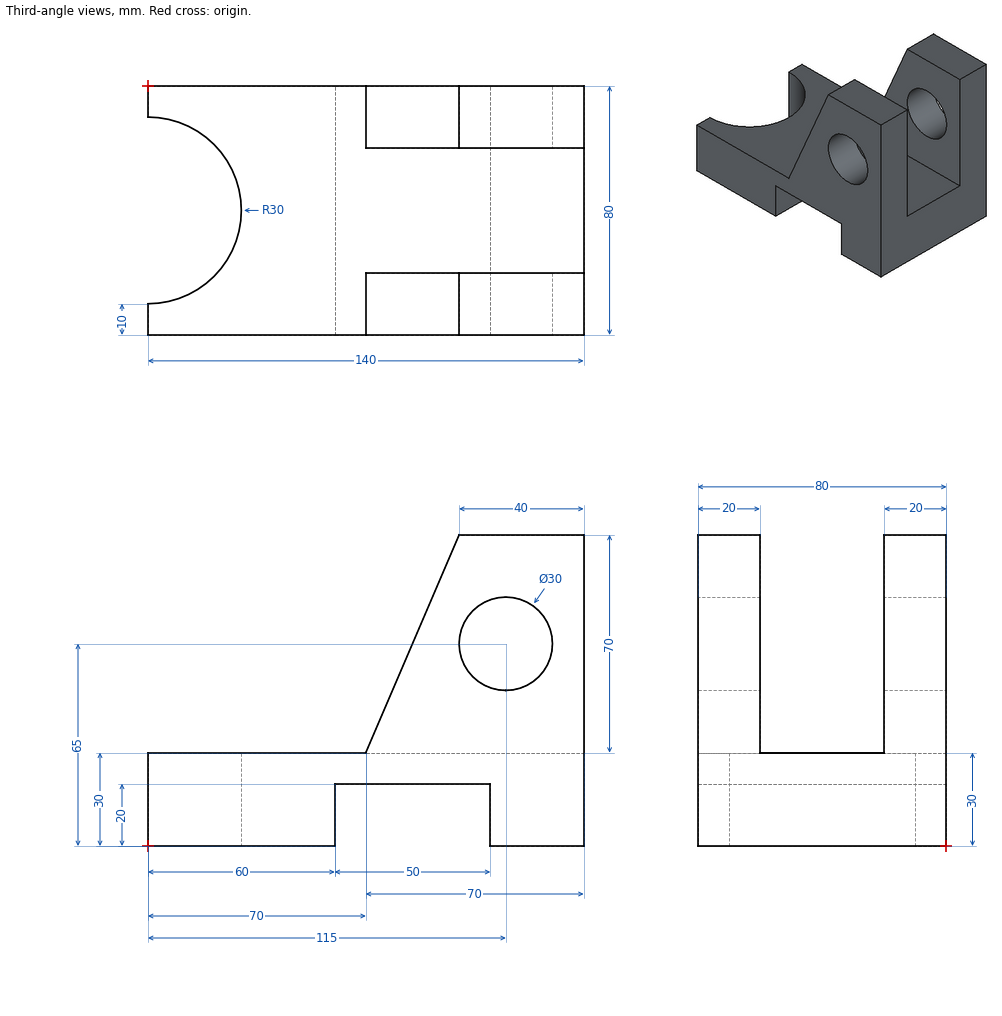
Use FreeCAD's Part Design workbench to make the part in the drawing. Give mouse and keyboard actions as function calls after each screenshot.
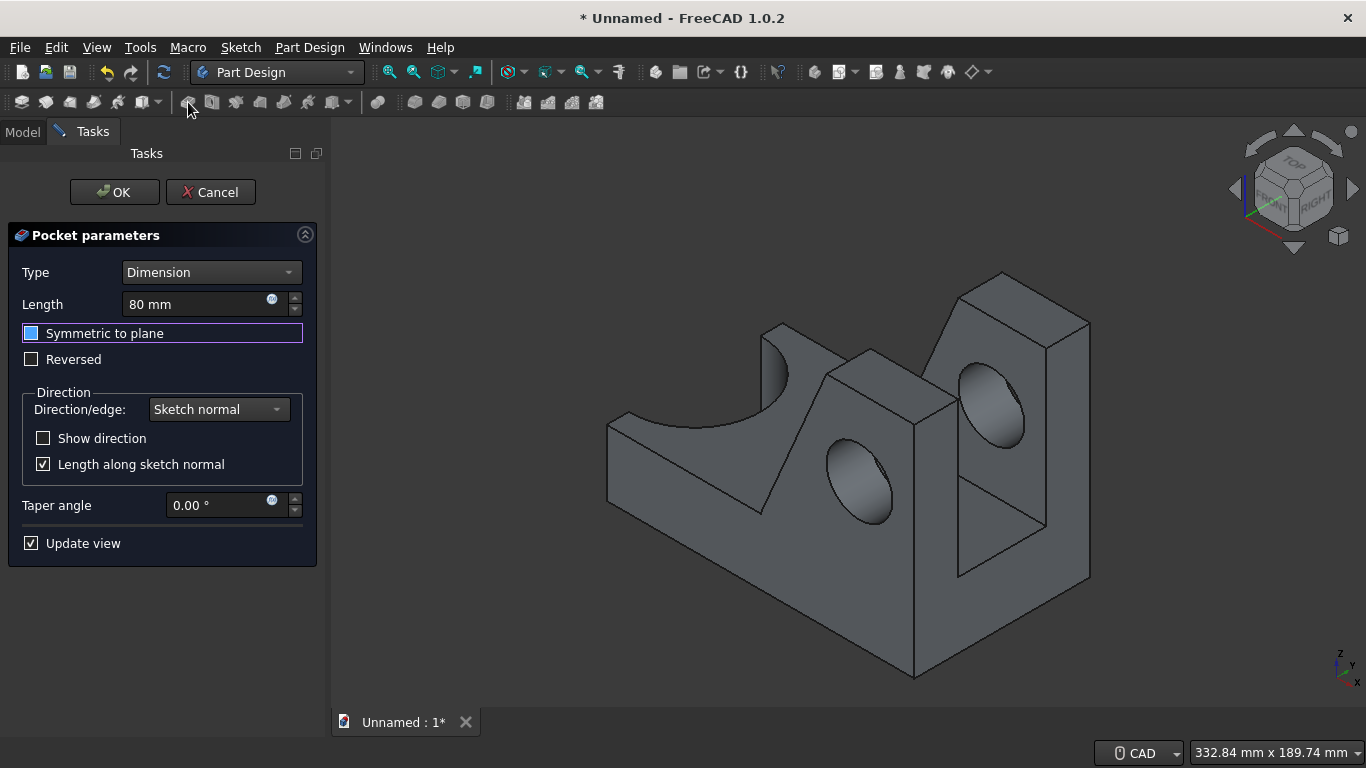
click(115, 192)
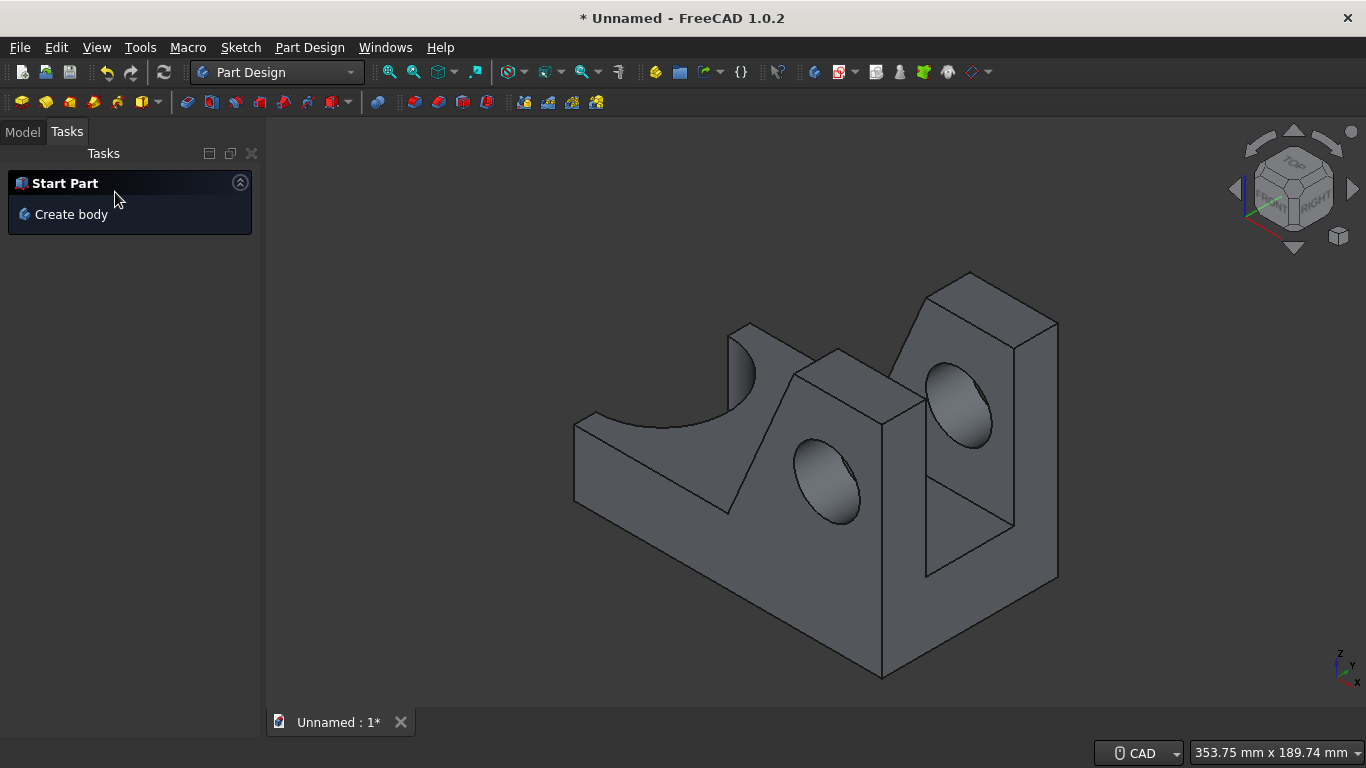
click(816, 585)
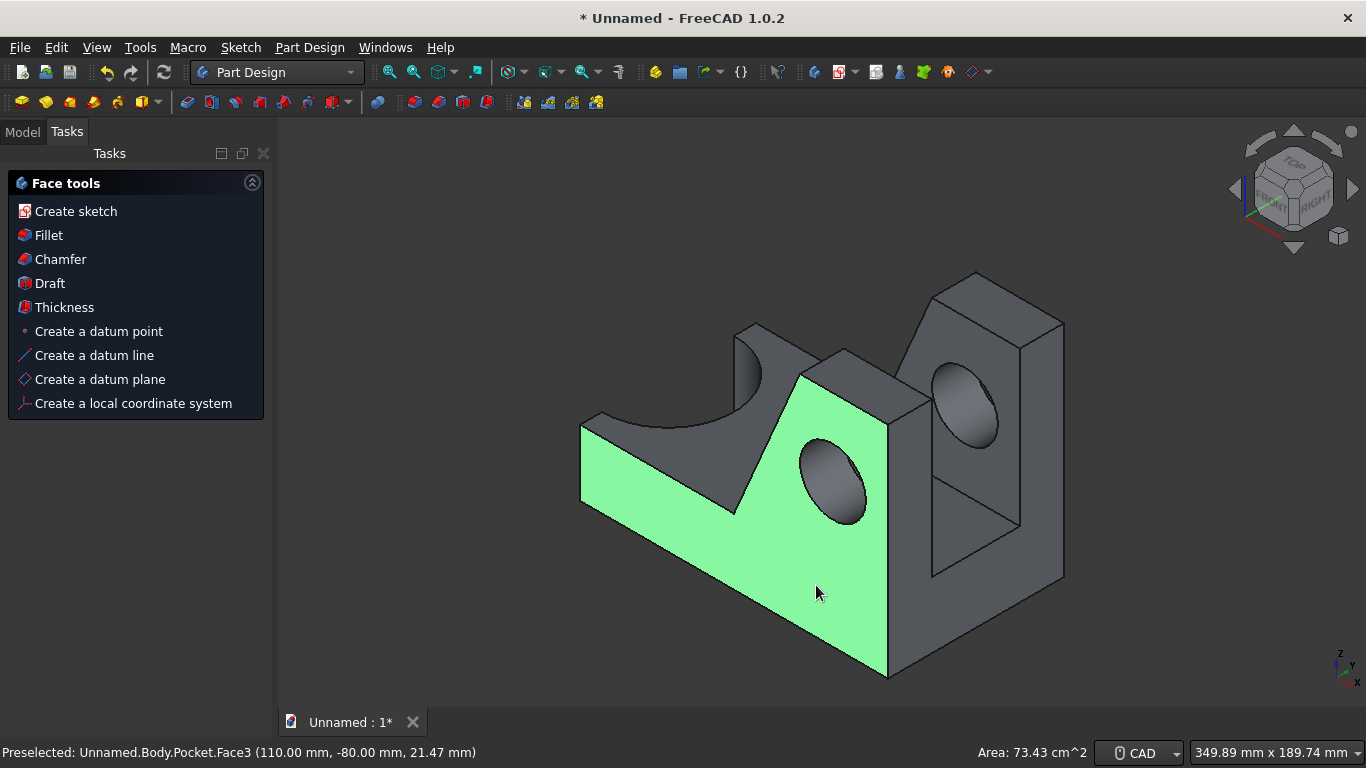
click(840, 72)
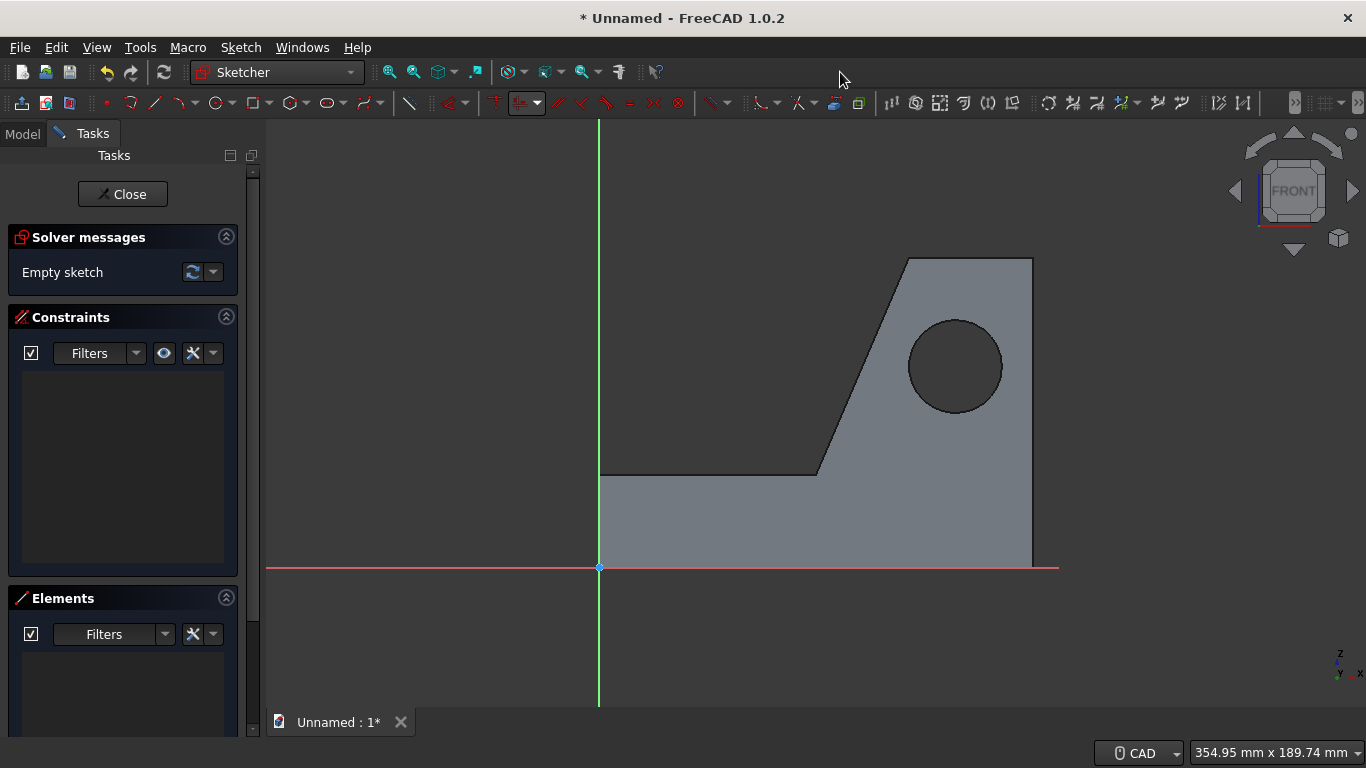
scroll(796, 679, up, 3)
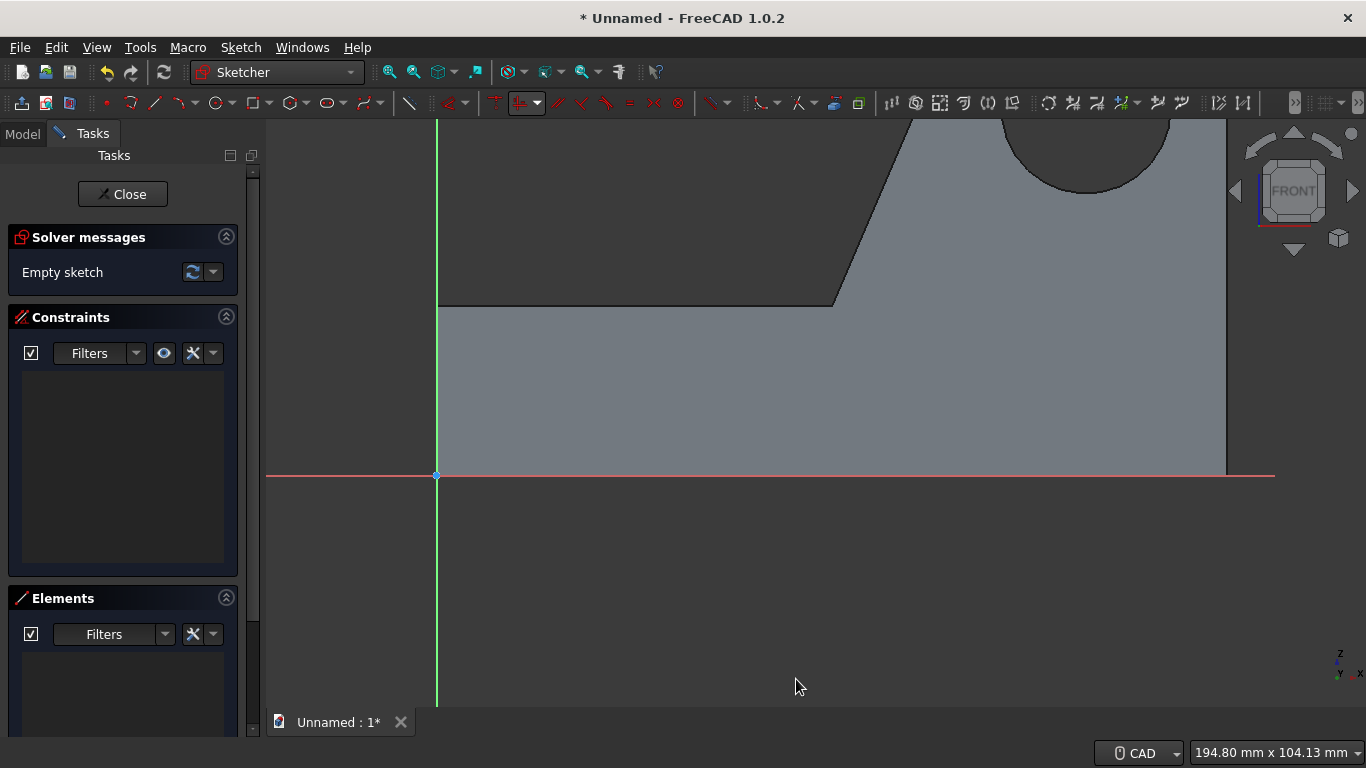
click(254, 104)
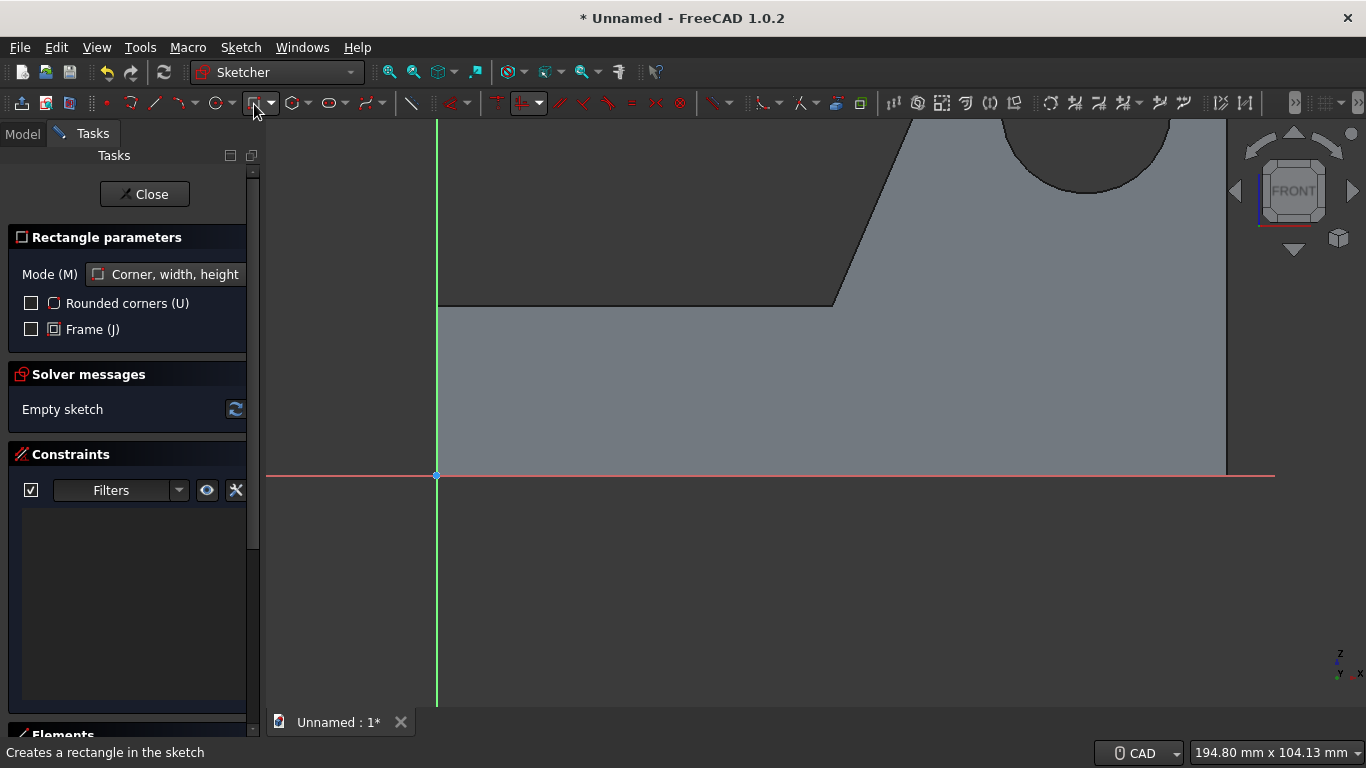
click(776, 363)
click(1058, 476)
key(Escape)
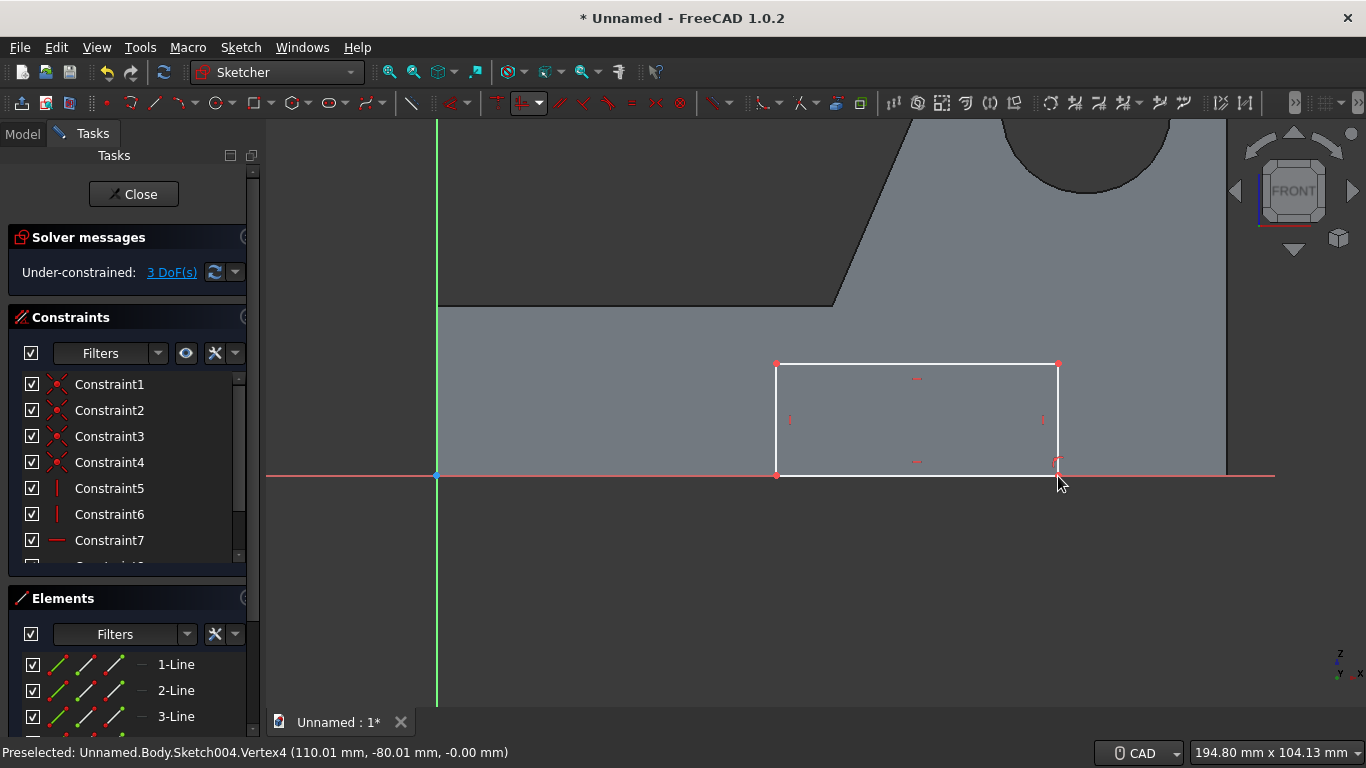
click(450, 104)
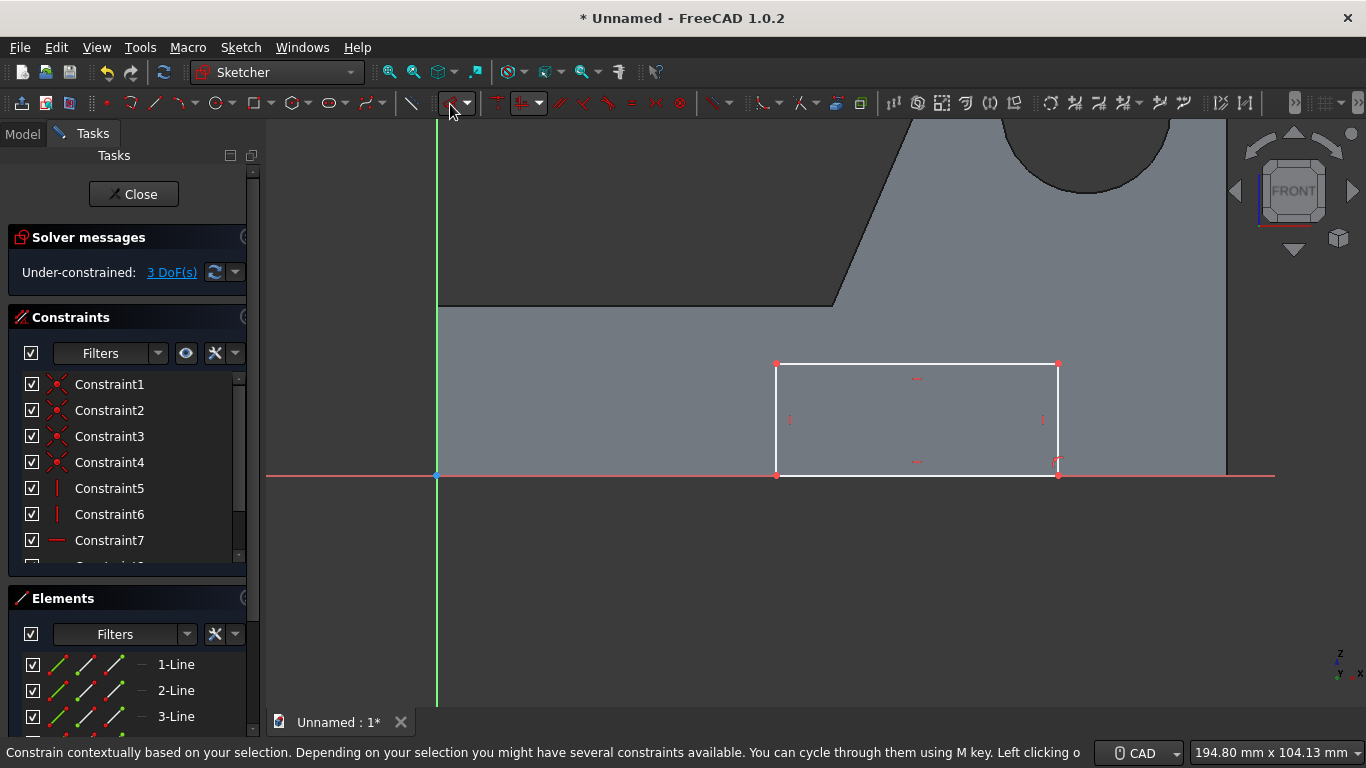
click(776, 398)
click(810, 420)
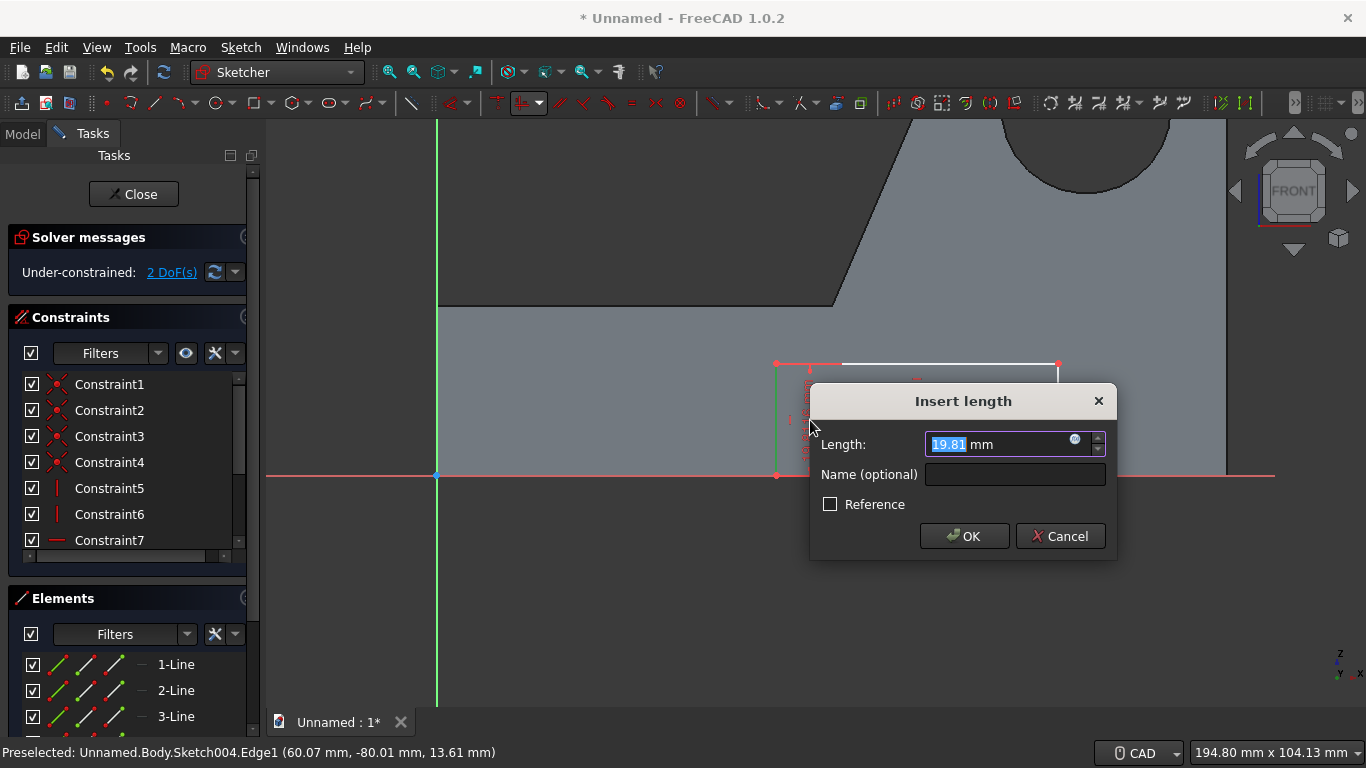
text(20)
key(Return)